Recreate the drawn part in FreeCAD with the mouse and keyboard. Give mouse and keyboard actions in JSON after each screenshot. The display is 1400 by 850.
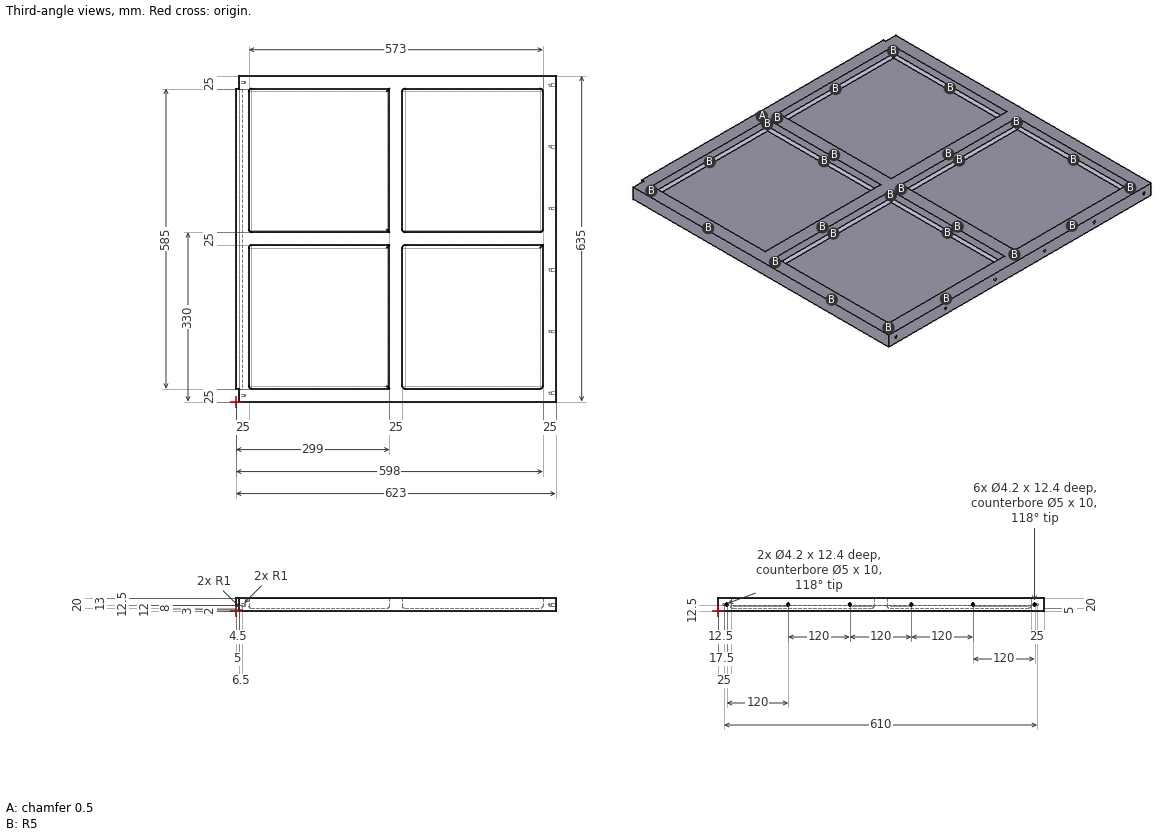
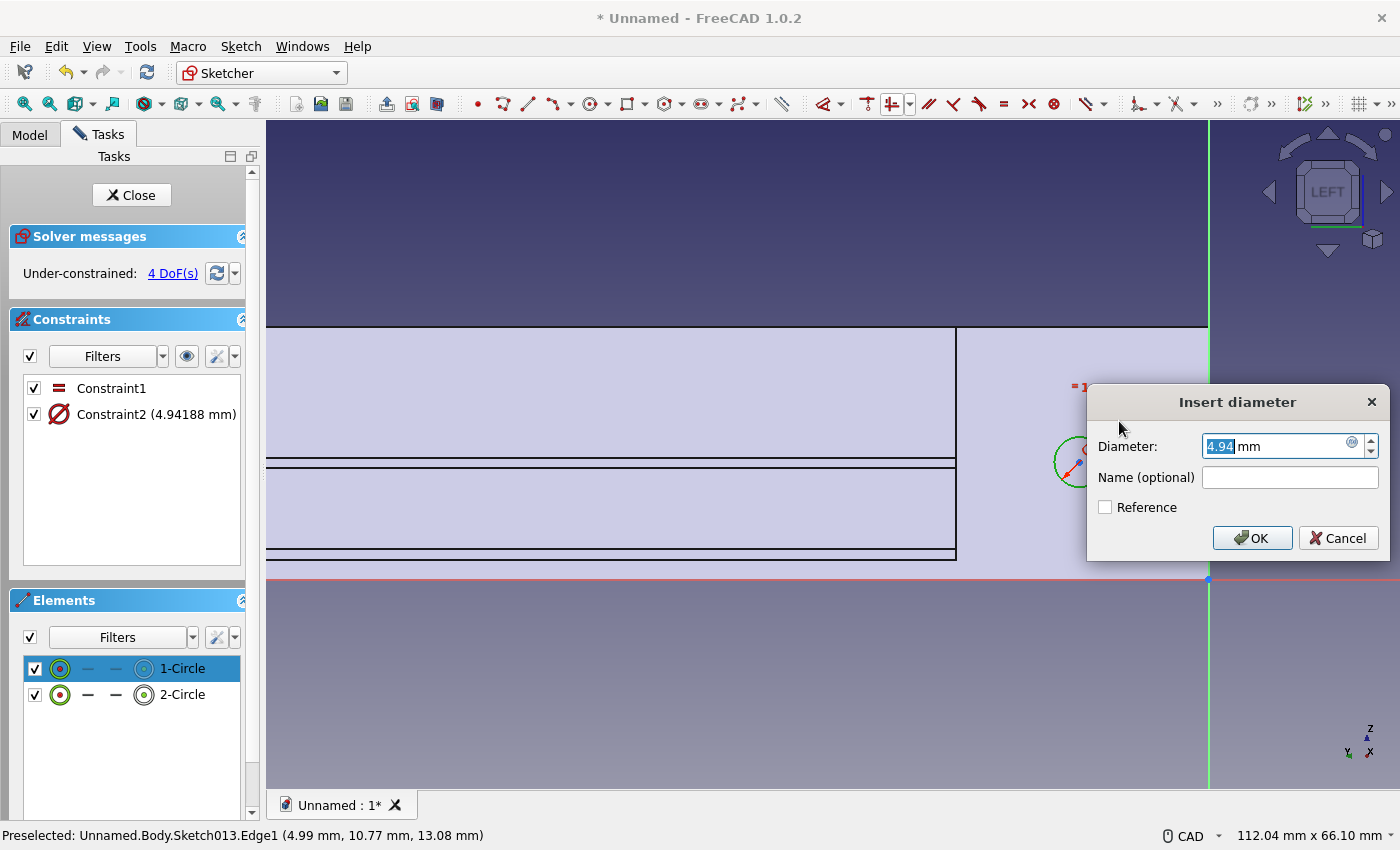
{"action": "type", "text": "4.2"}
{"action": "key", "text": "Return"}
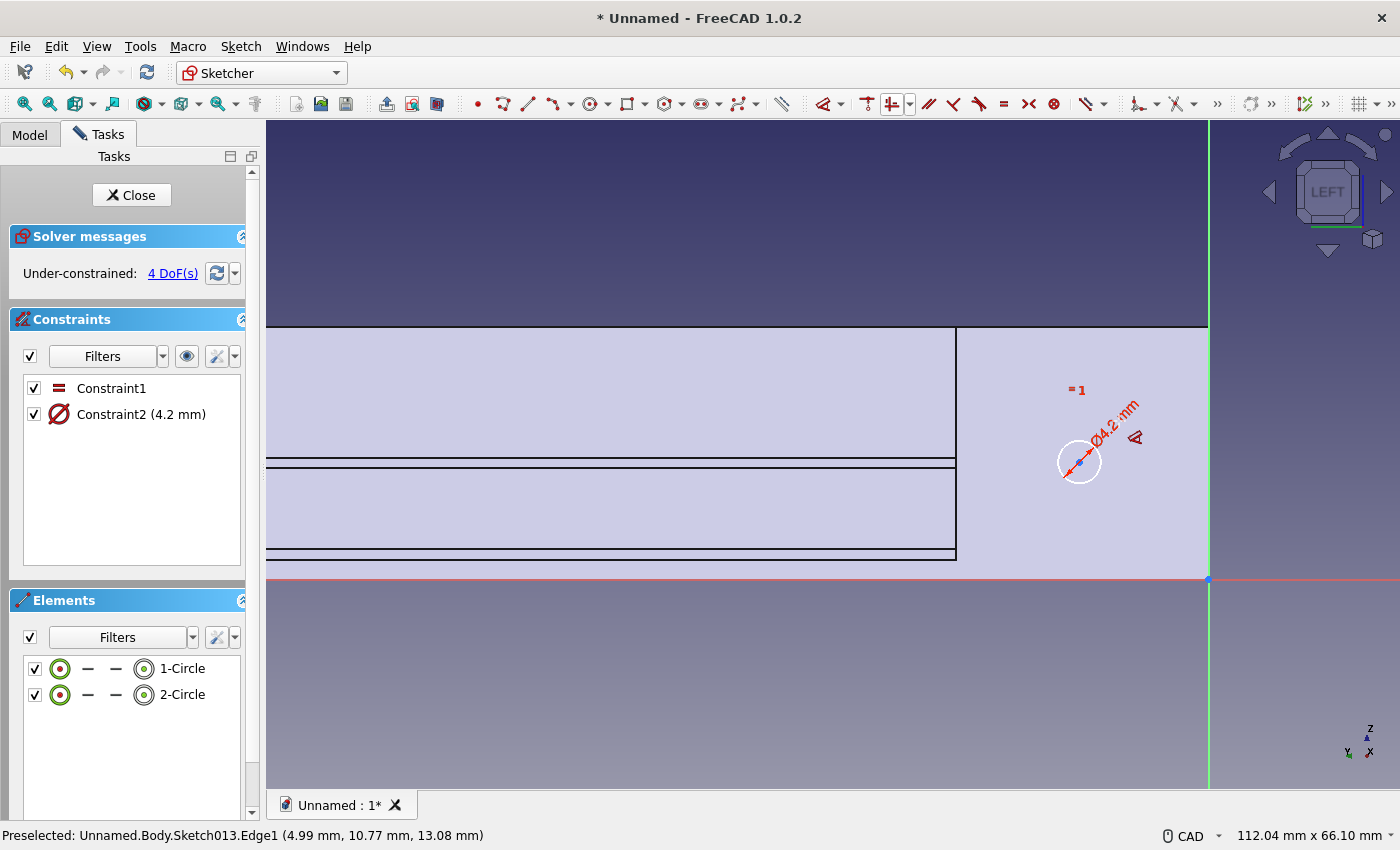
{"action": "scroll", "coordinate": [1103, 448], "scroll_direction": "down", "scroll_amount": 11}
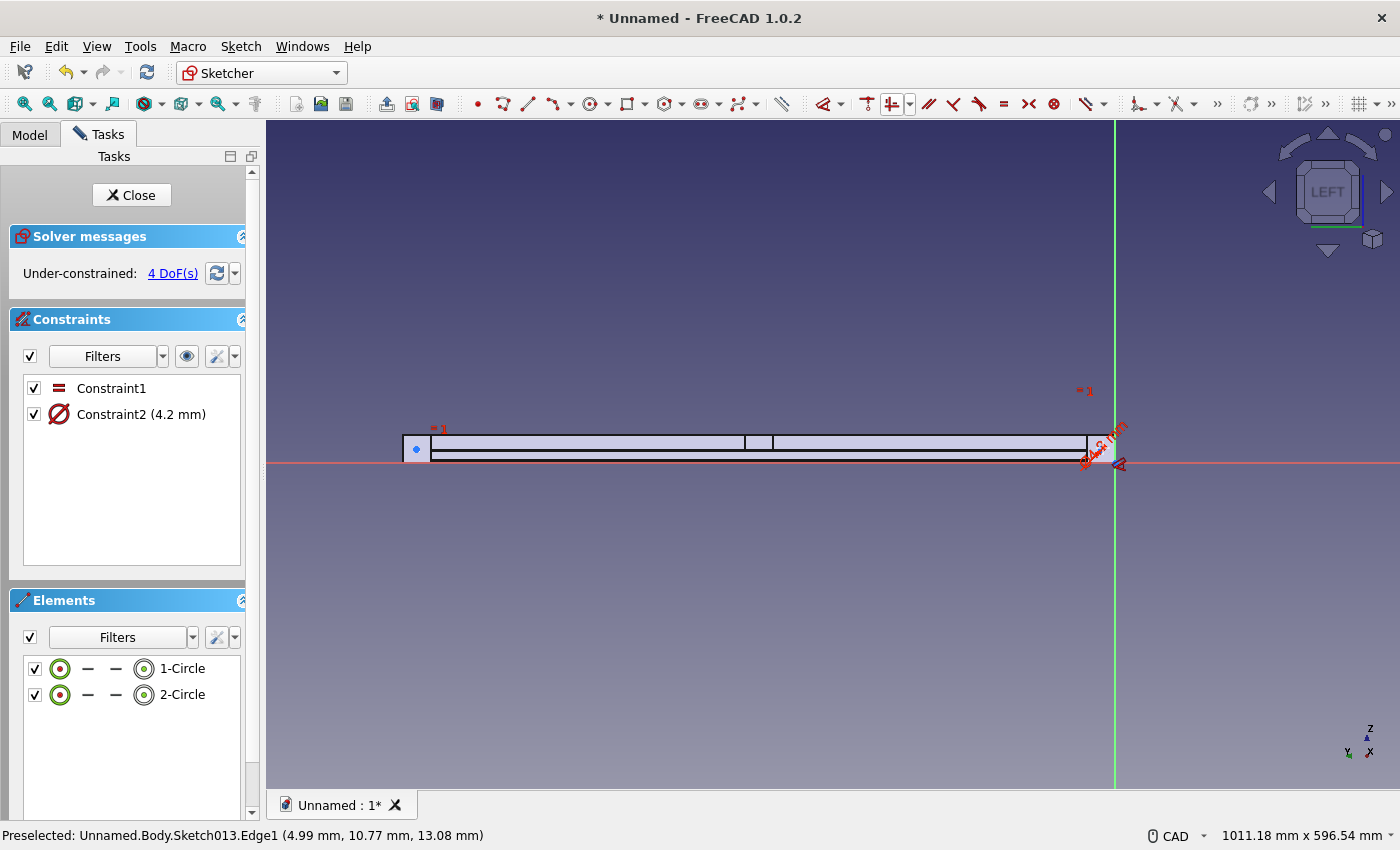
{"action": "scroll", "coordinate": [1101, 450], "scroll_direction": "up", "scroll_amount": 6}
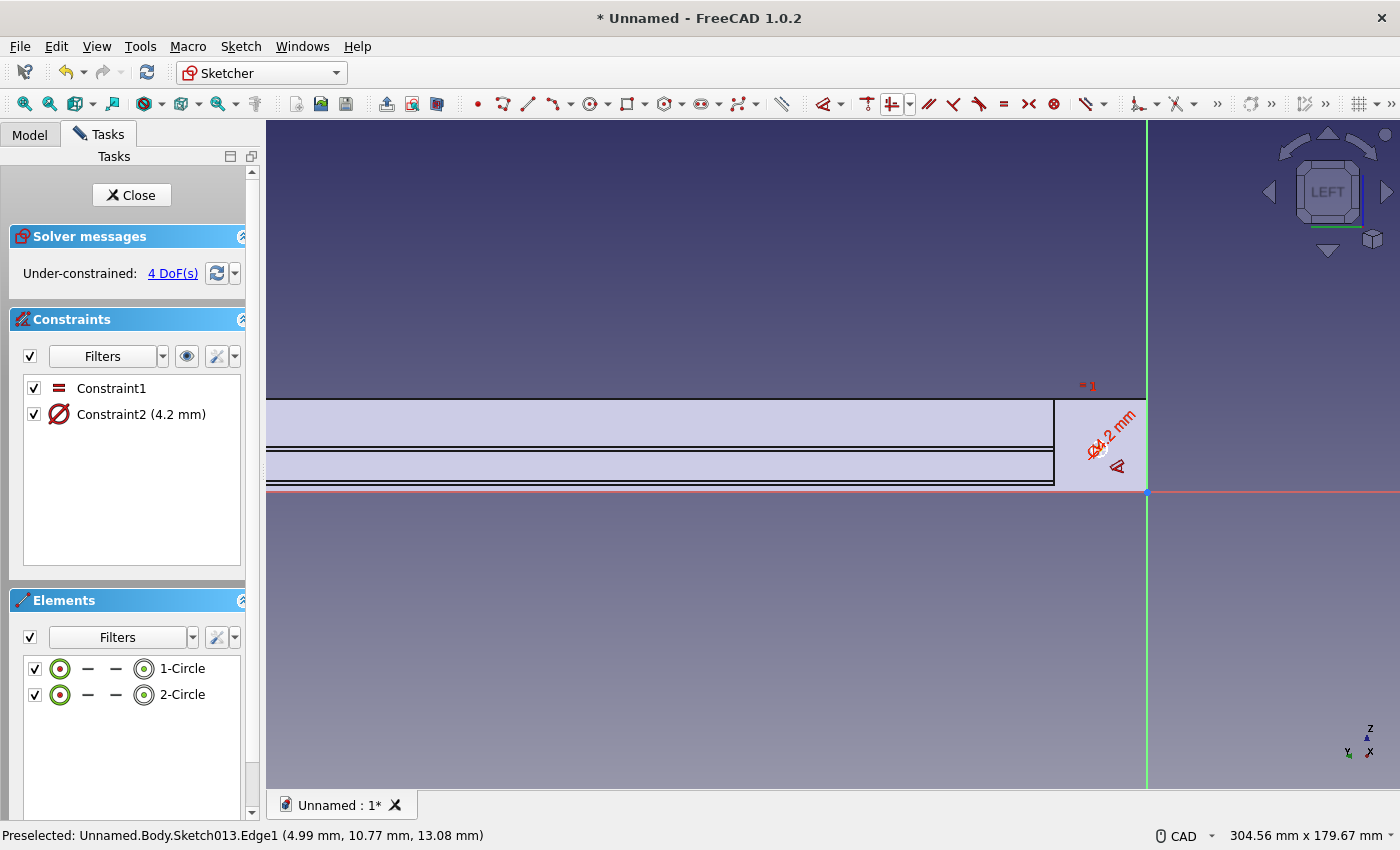
{"action": "left_click", "coordinate": [1099, 449]}
{"action": "left_click", "coordinate": [1123, 526]}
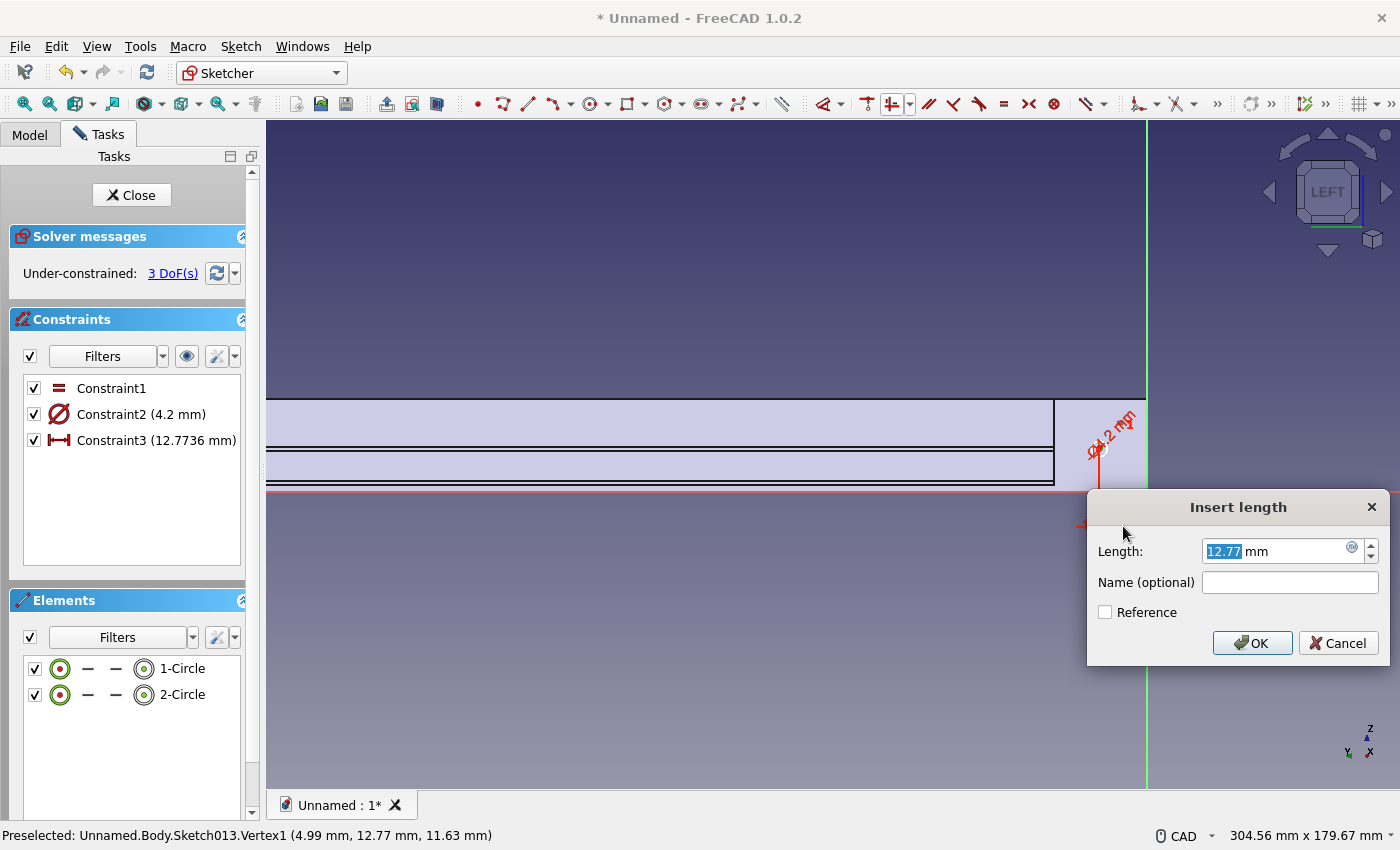
{"action": "type", "text": "12.5"}
{"action": "key", "text": "Return"}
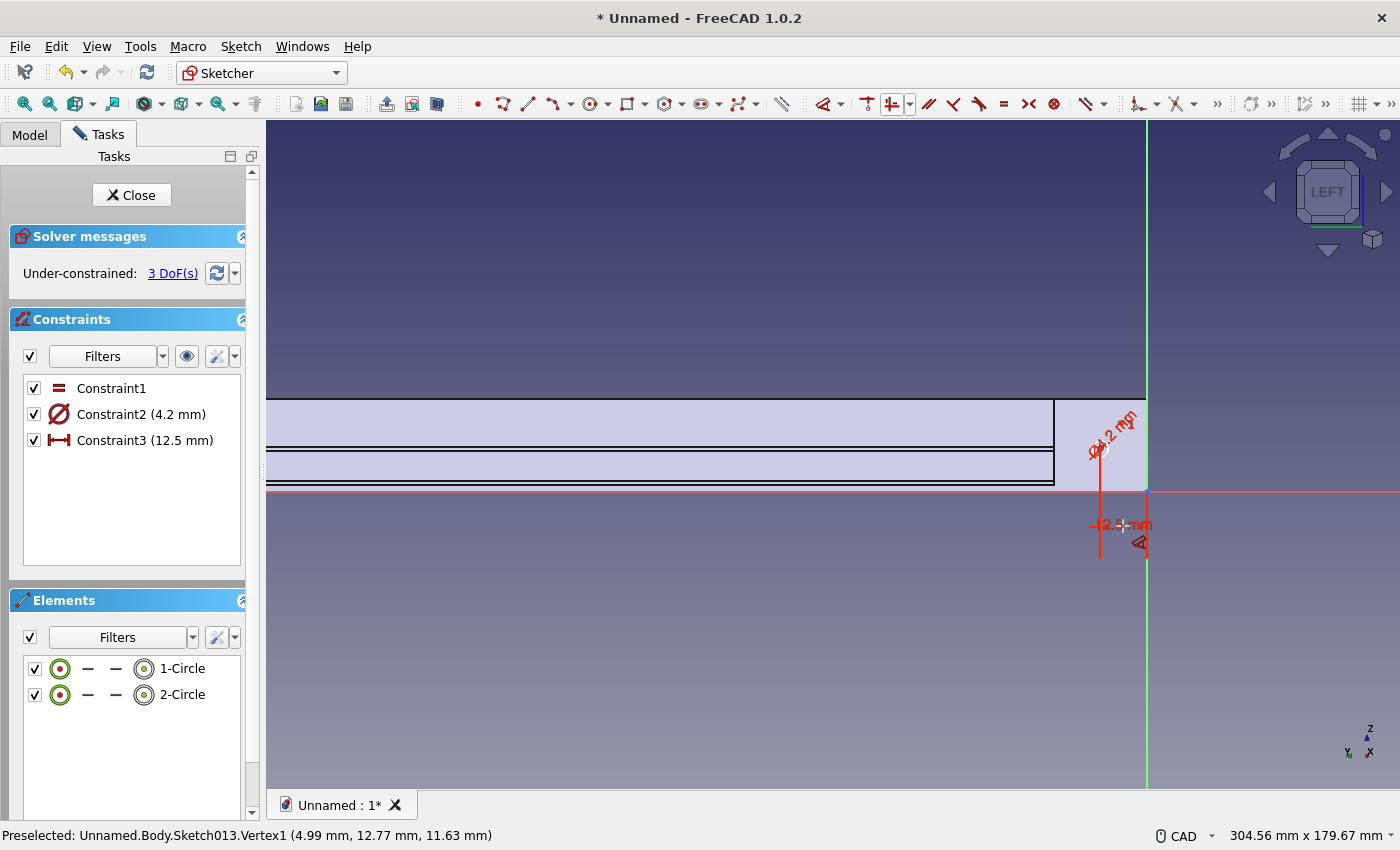
{"action": "left_click", "coordinate": [1100, 449]}
{"action": "left_click", "coordinate": [1181, 471]}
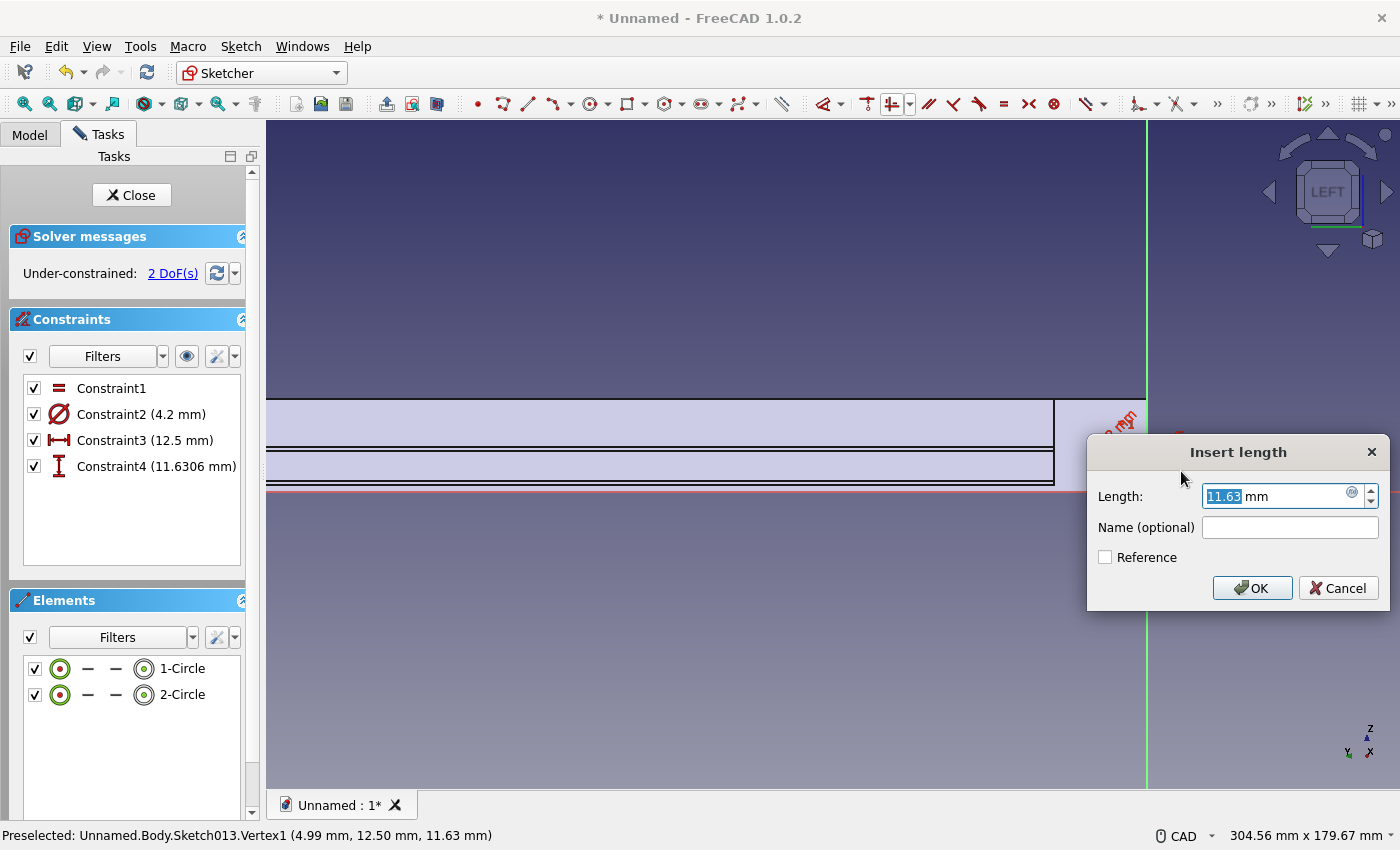
{"action": "type", "text": "12.5"}
{"action": "key", "text": "Return"}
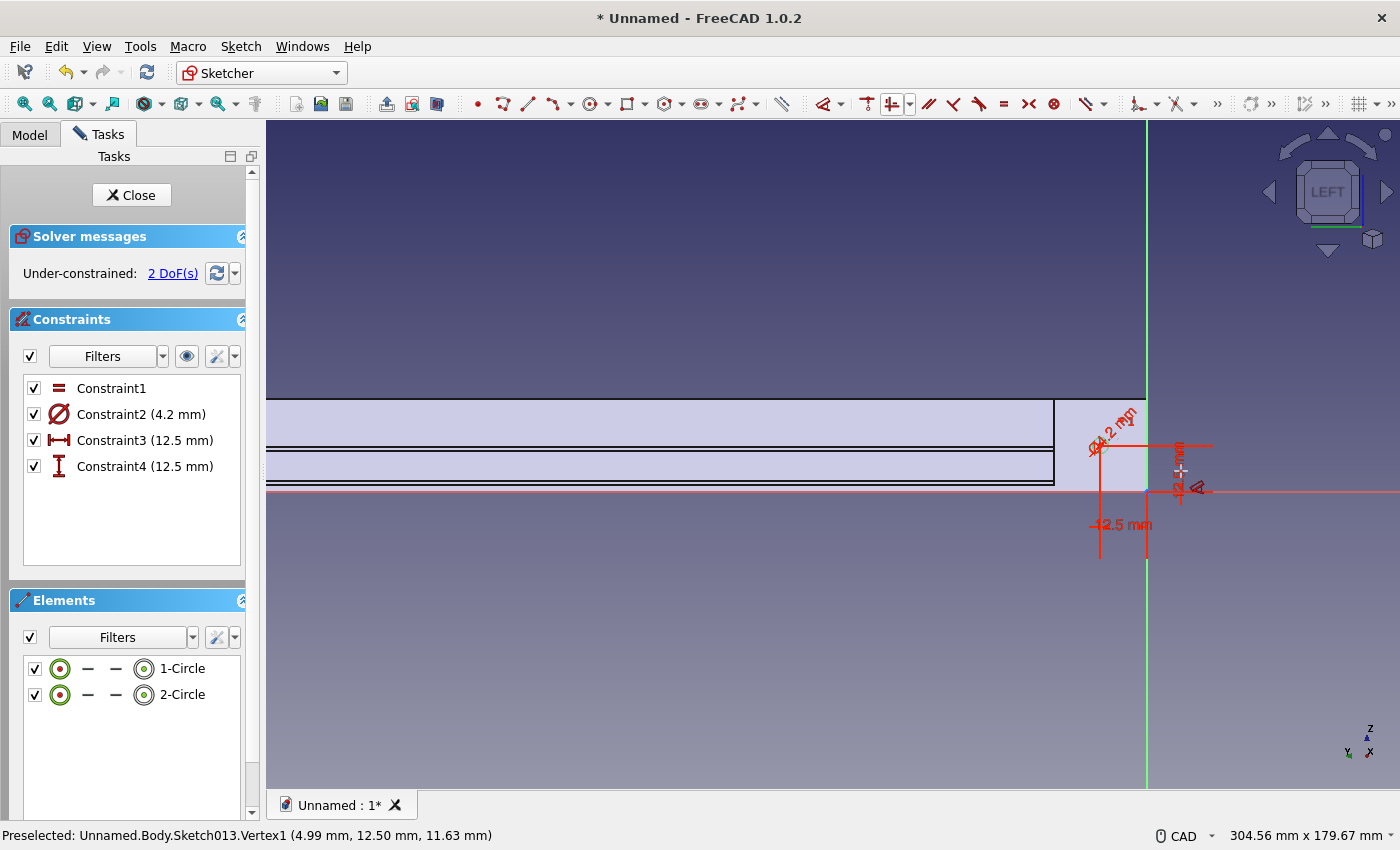
{"action": "scroll", "coordinate": [1101, 450], "scroll_direction": "down", "scroll_amount": 6}